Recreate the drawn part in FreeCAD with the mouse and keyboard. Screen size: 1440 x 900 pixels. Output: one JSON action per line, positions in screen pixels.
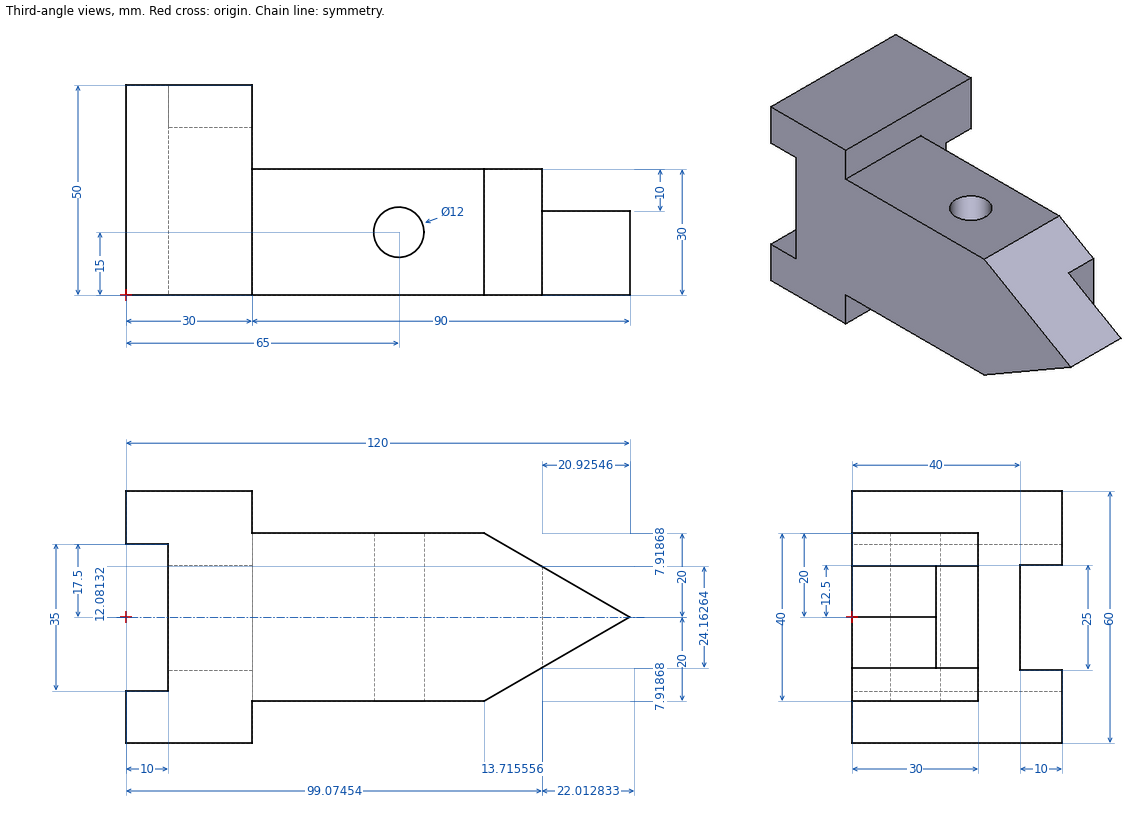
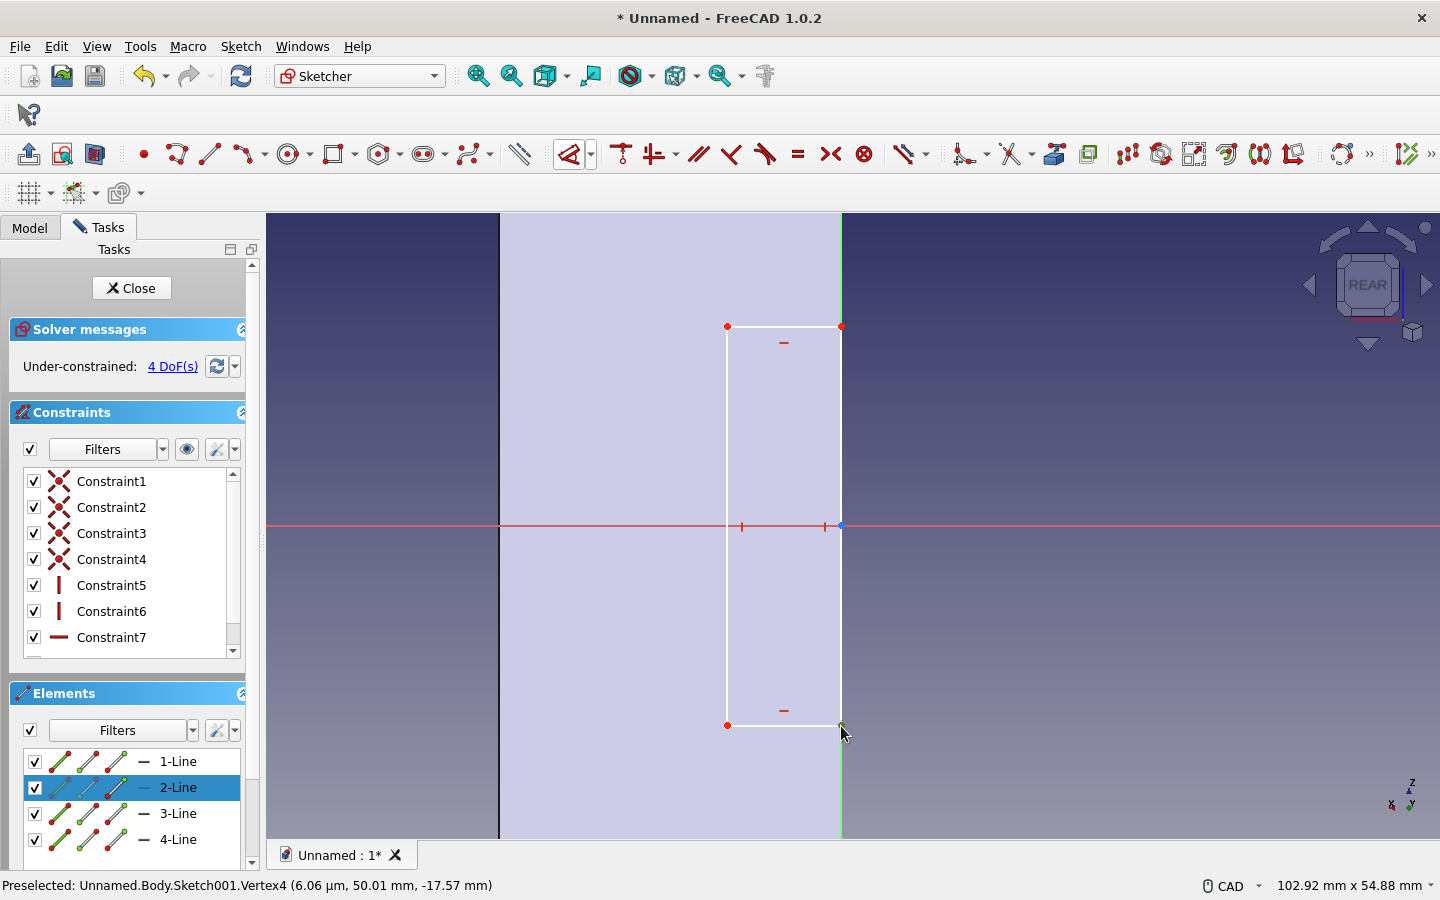
{"action": "left_click", "coordinate": [841, 770]}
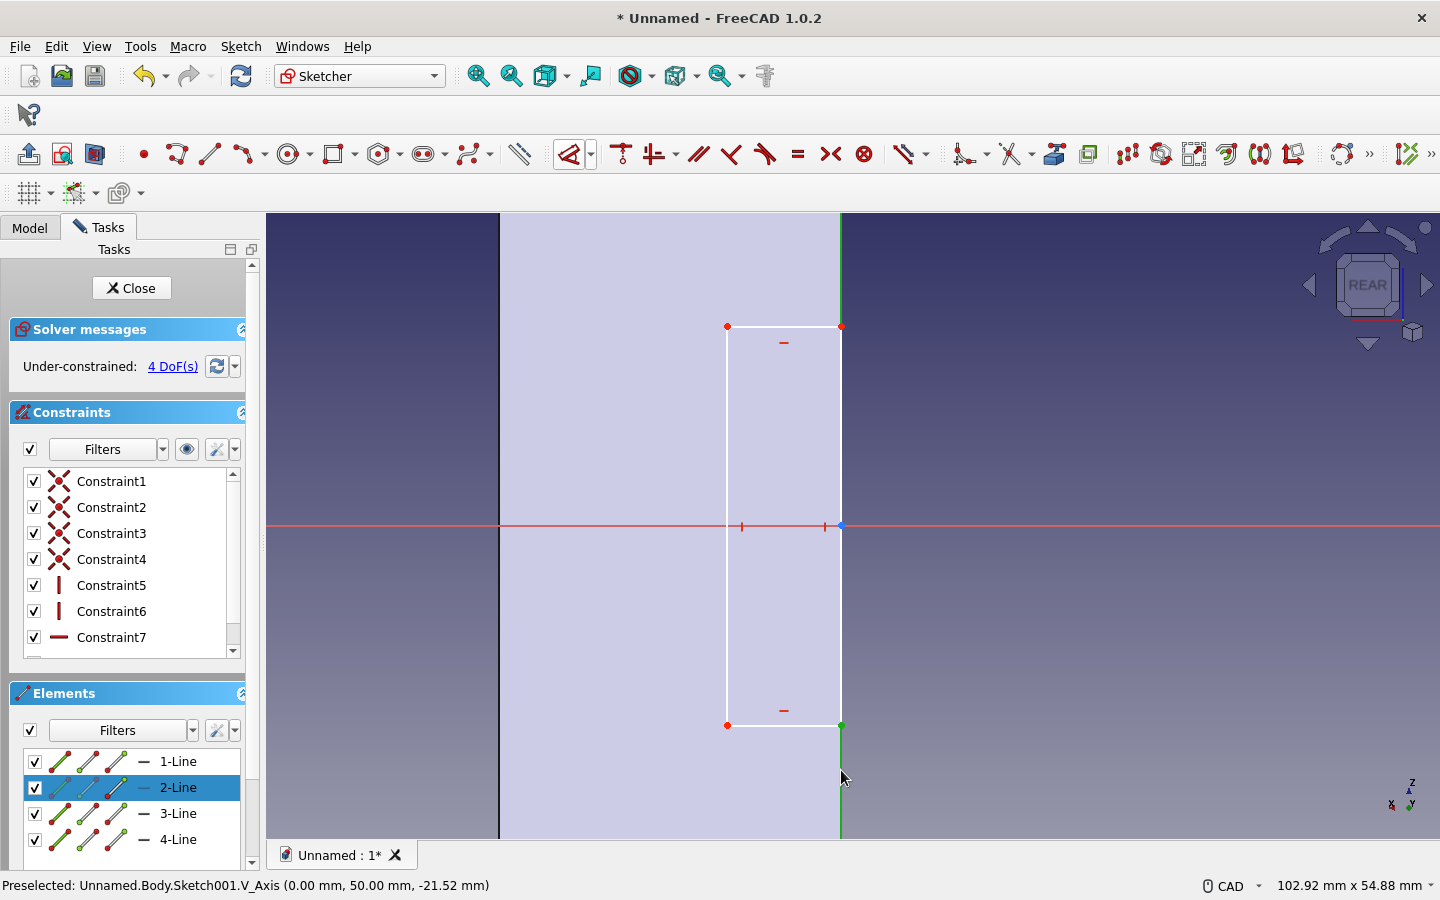
{"action": "left_click", "coordinate": [621, 154]}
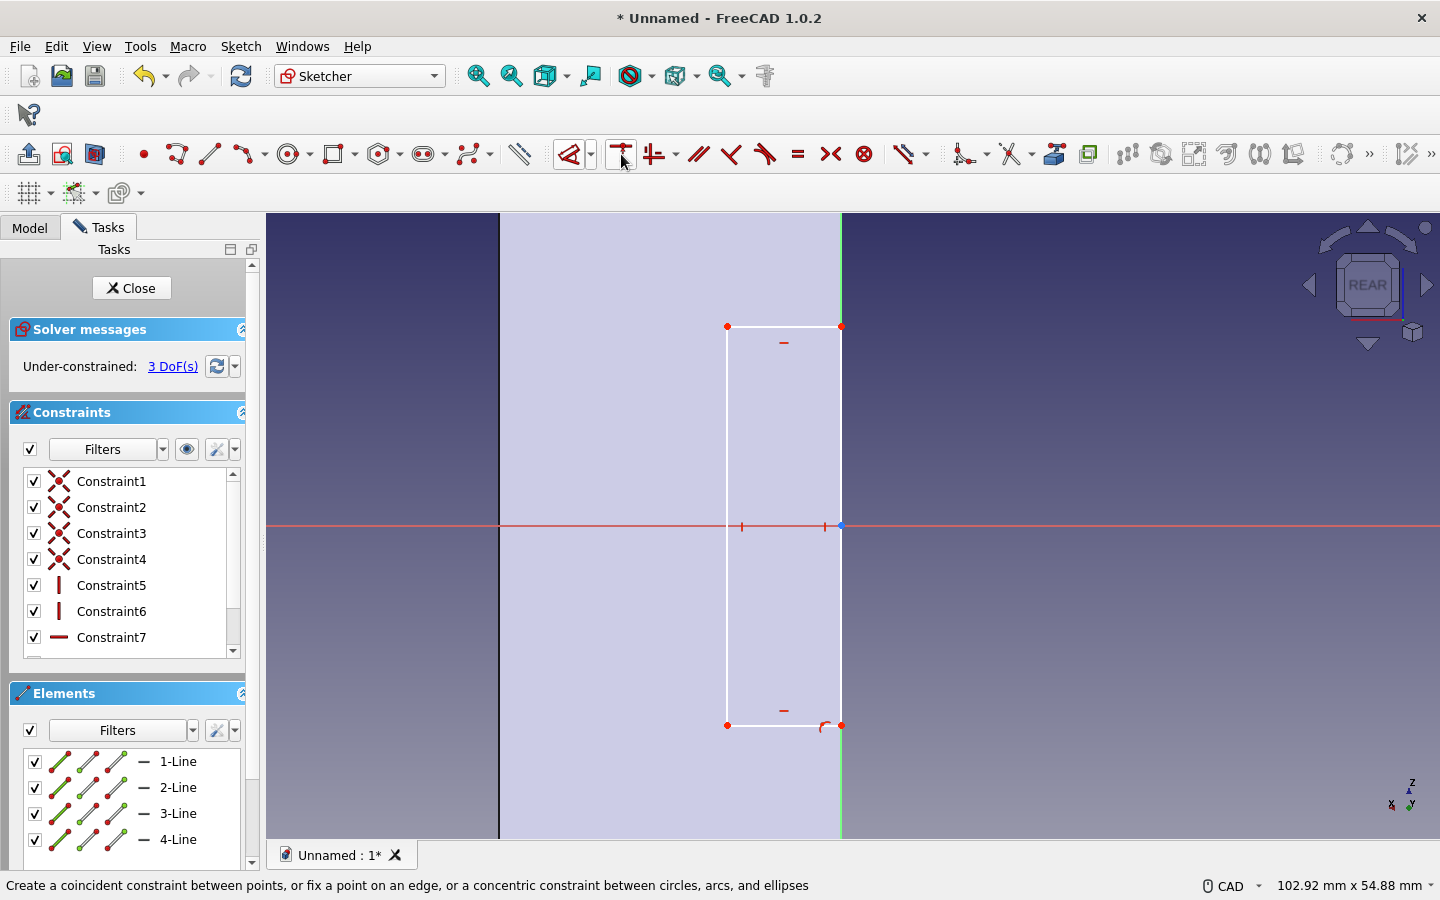
{"action": "left_click", "coordinate": [727, 447]}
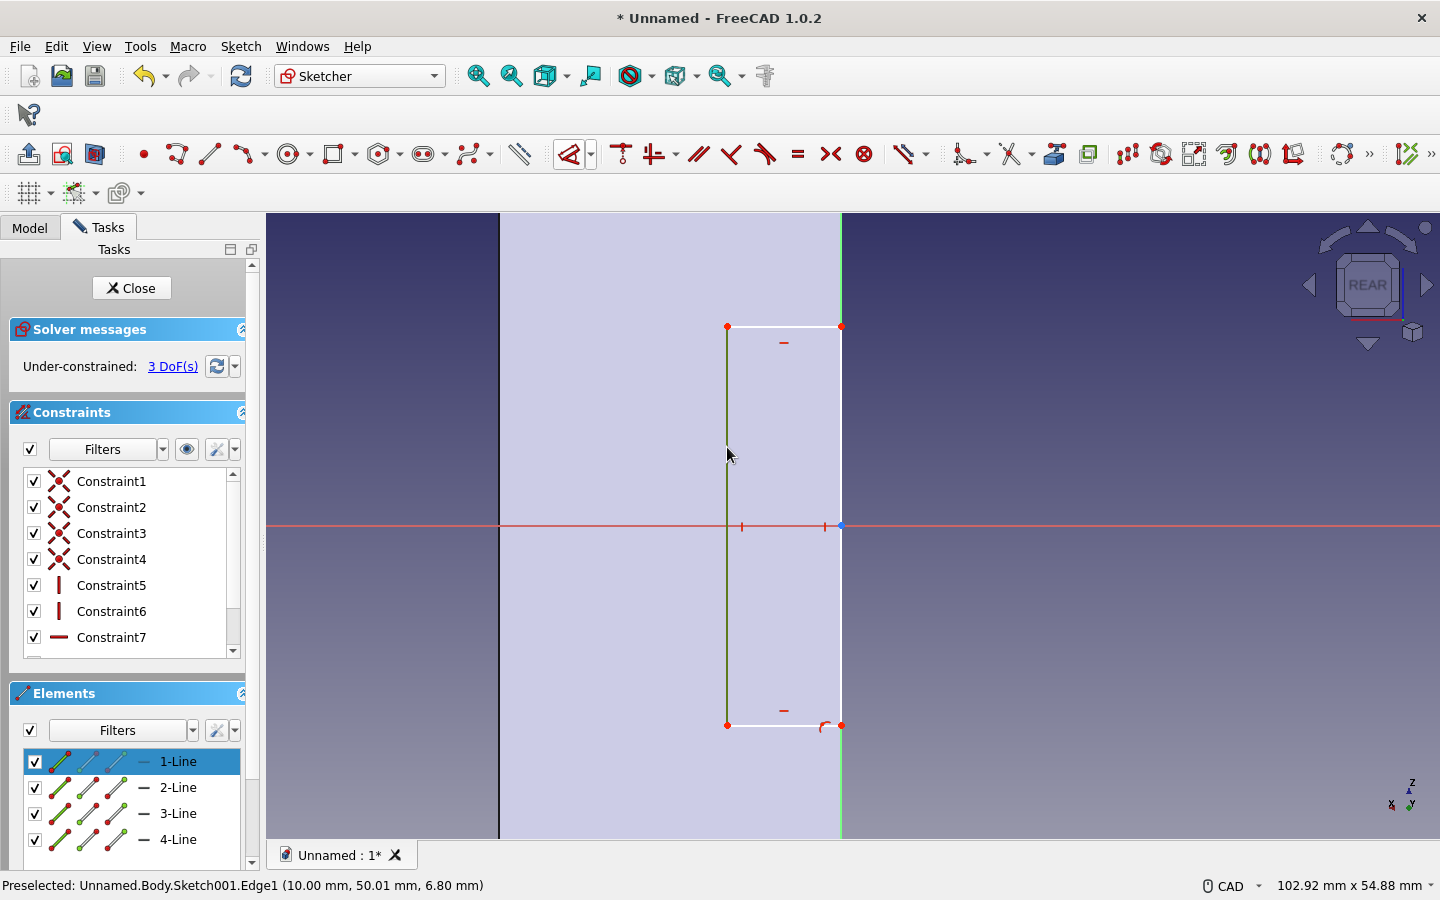
{"action": "key", "text": "i"}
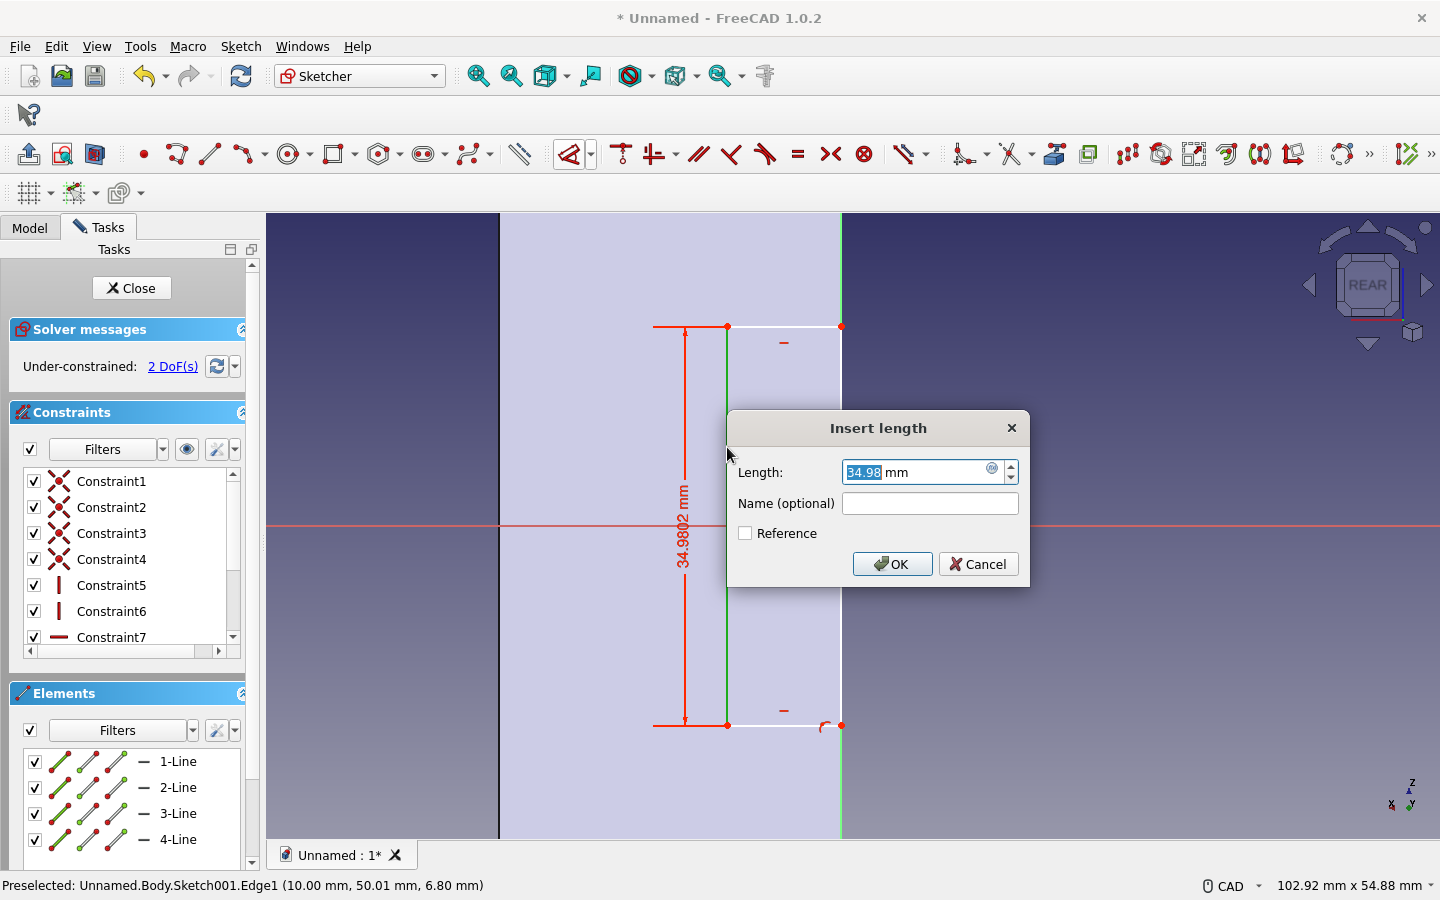
{"action": "type", "text": "35"}
{"action": "key", "text": "Return"}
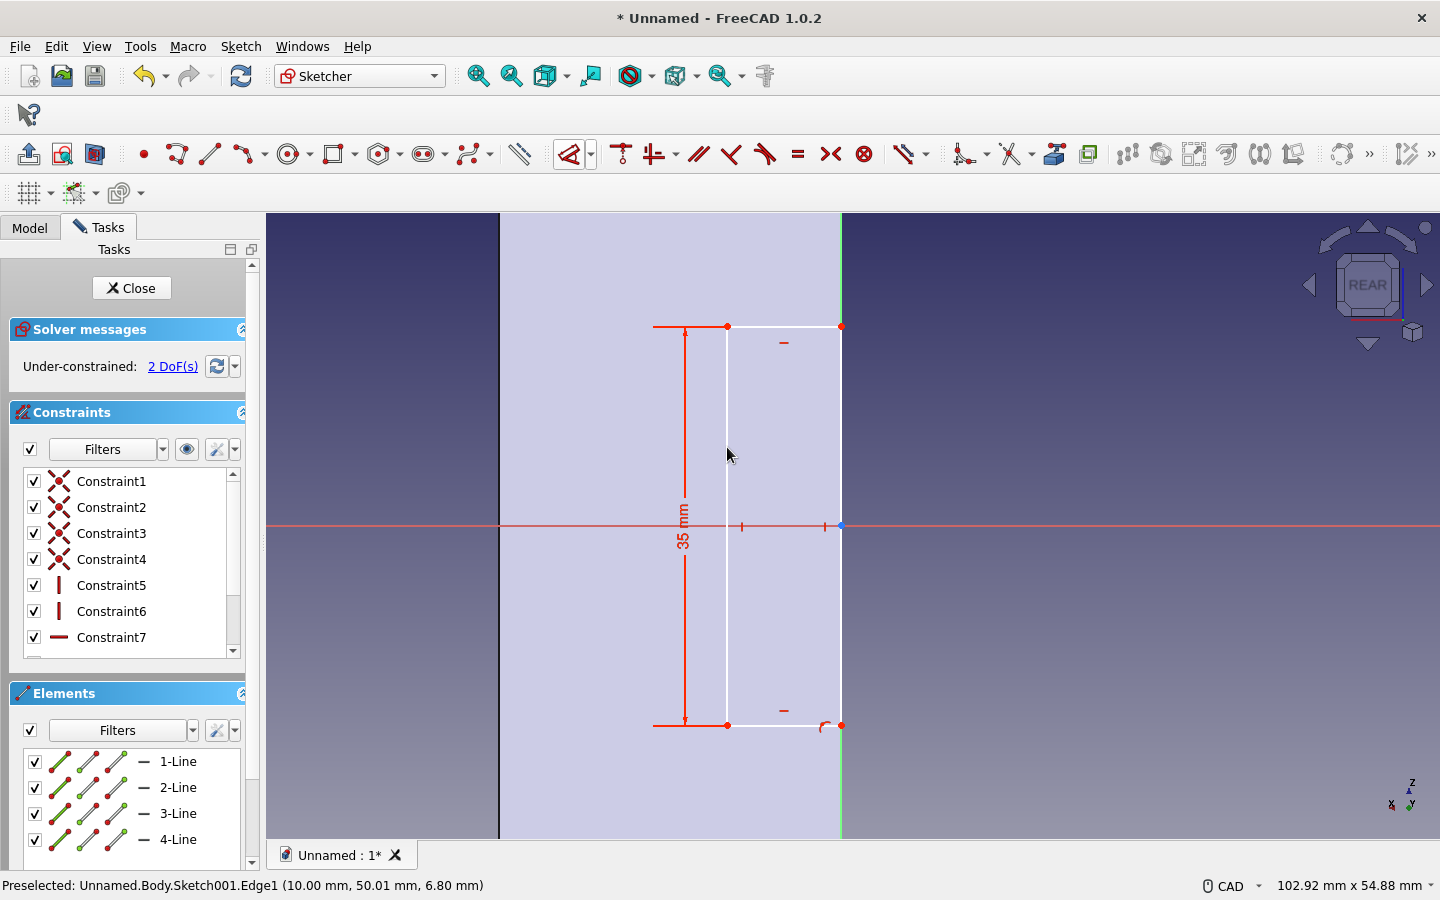
{"action": "left_click", "coordinate": [761, 726]}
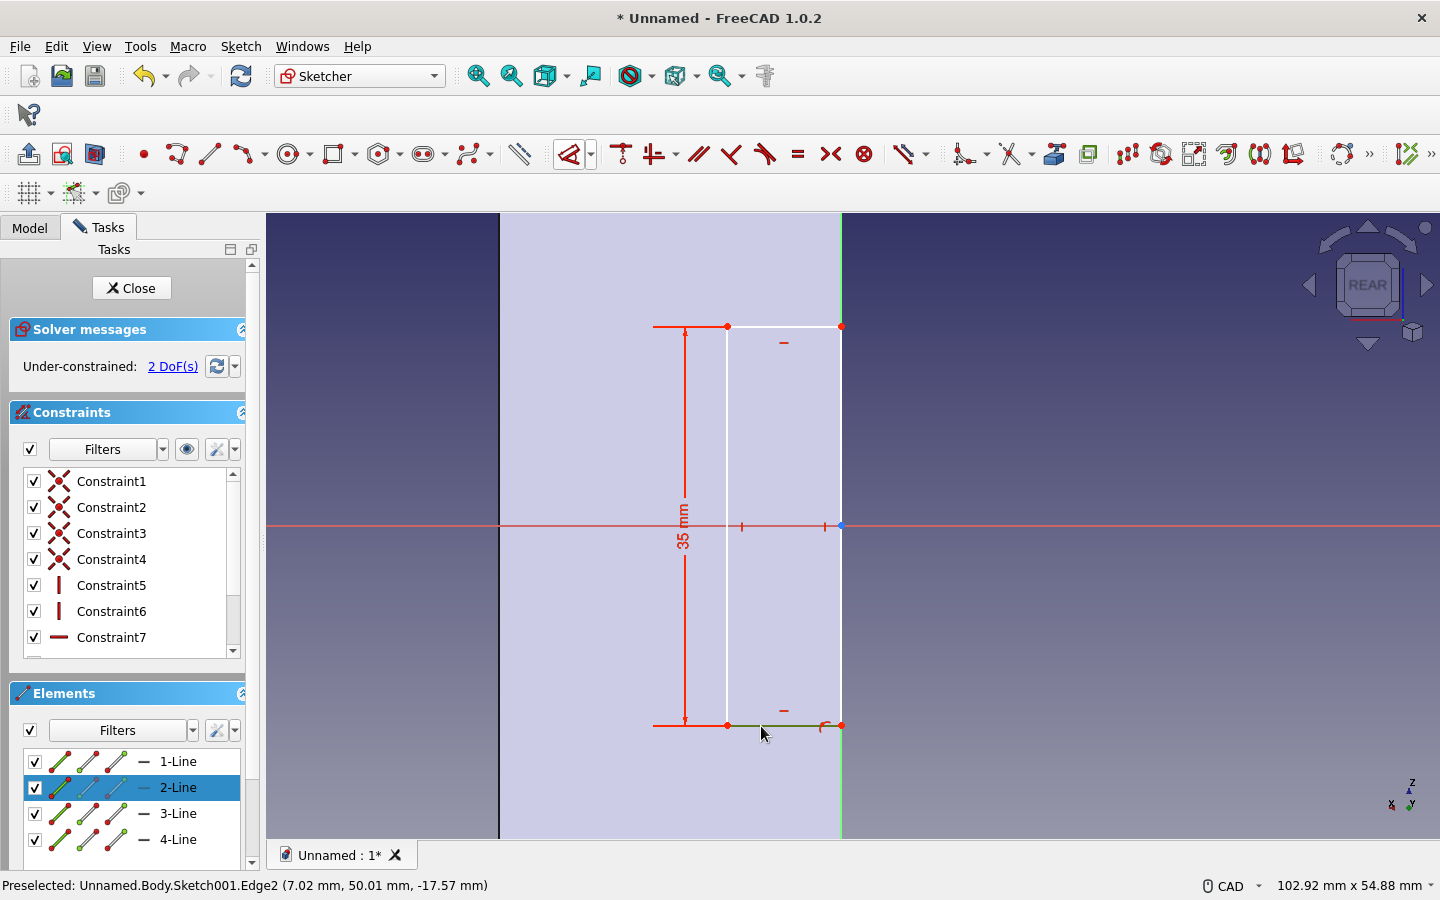
{"action": "key", "text": "l"}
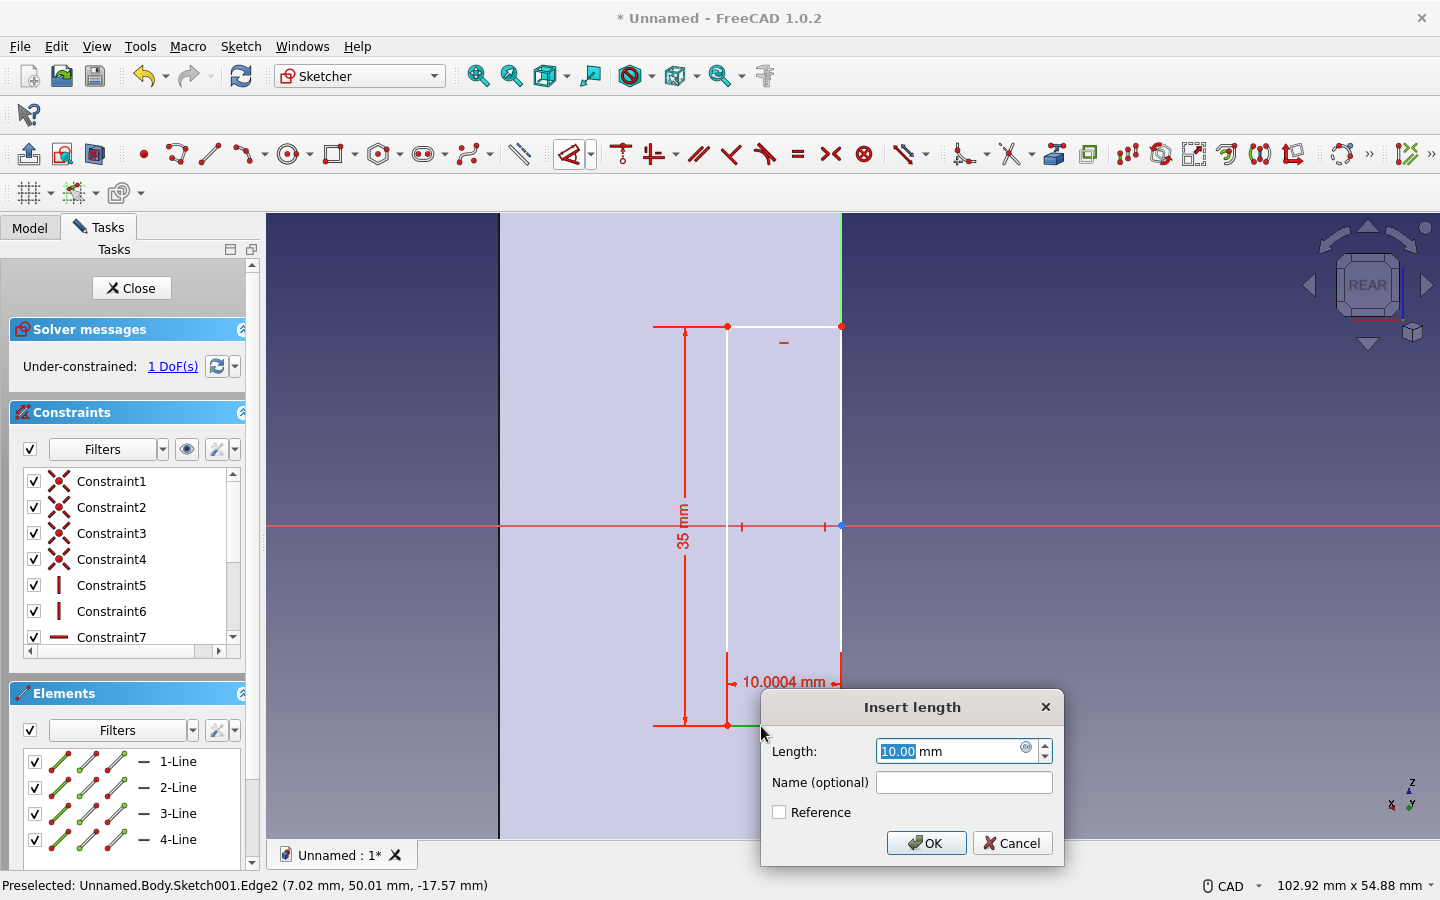
{"action": "type", "text": "10"}
{"action": "key", "text": "Return"}